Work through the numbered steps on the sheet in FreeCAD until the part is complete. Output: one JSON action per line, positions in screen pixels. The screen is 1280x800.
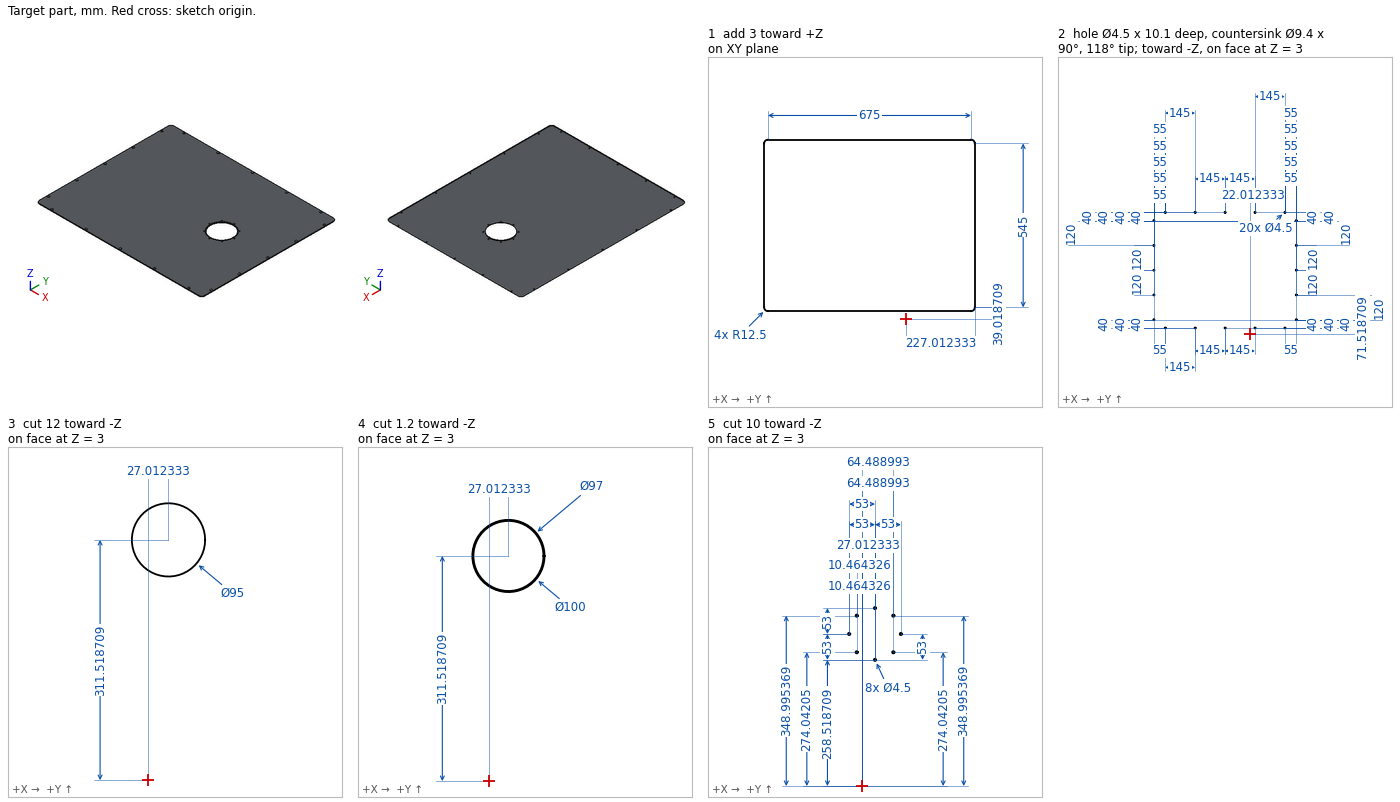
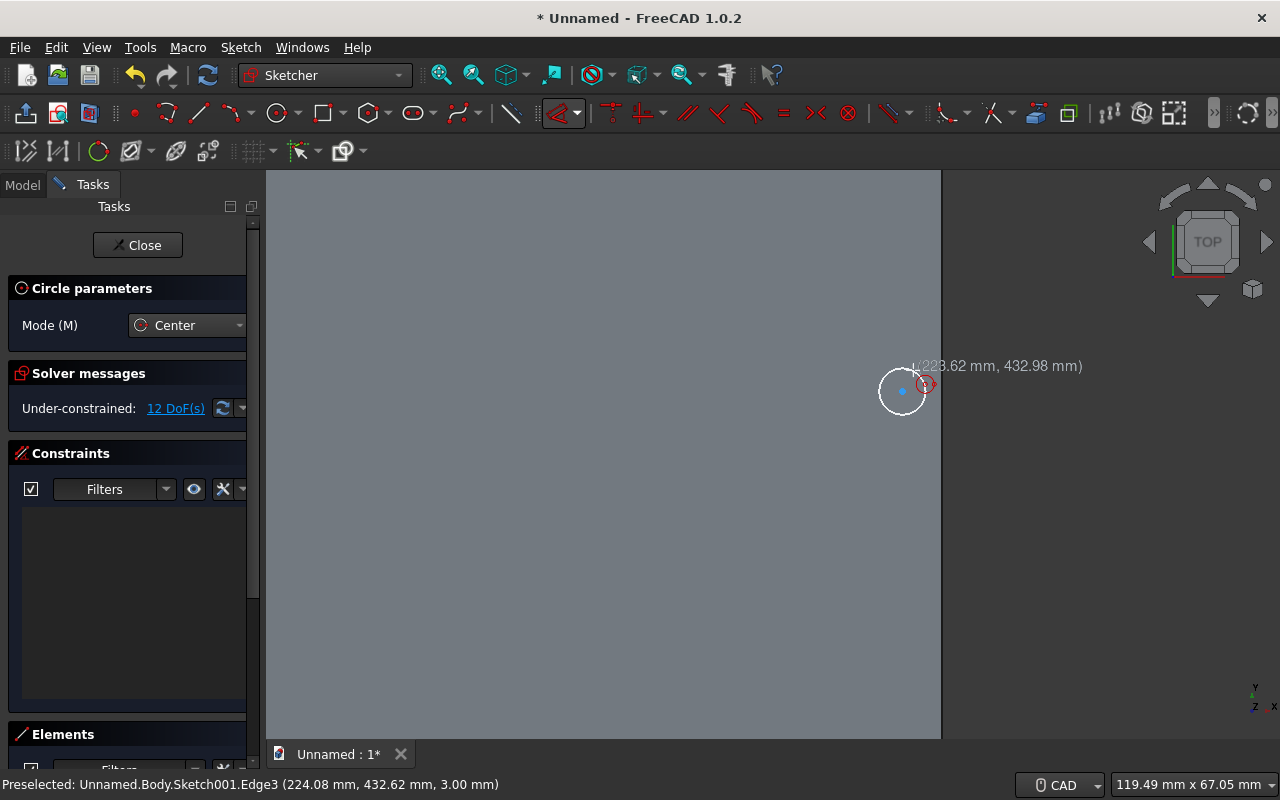
{"action": "scroll", "coordinate": [924, 369], "scroll_direction": "down", "scroll_amount": 13}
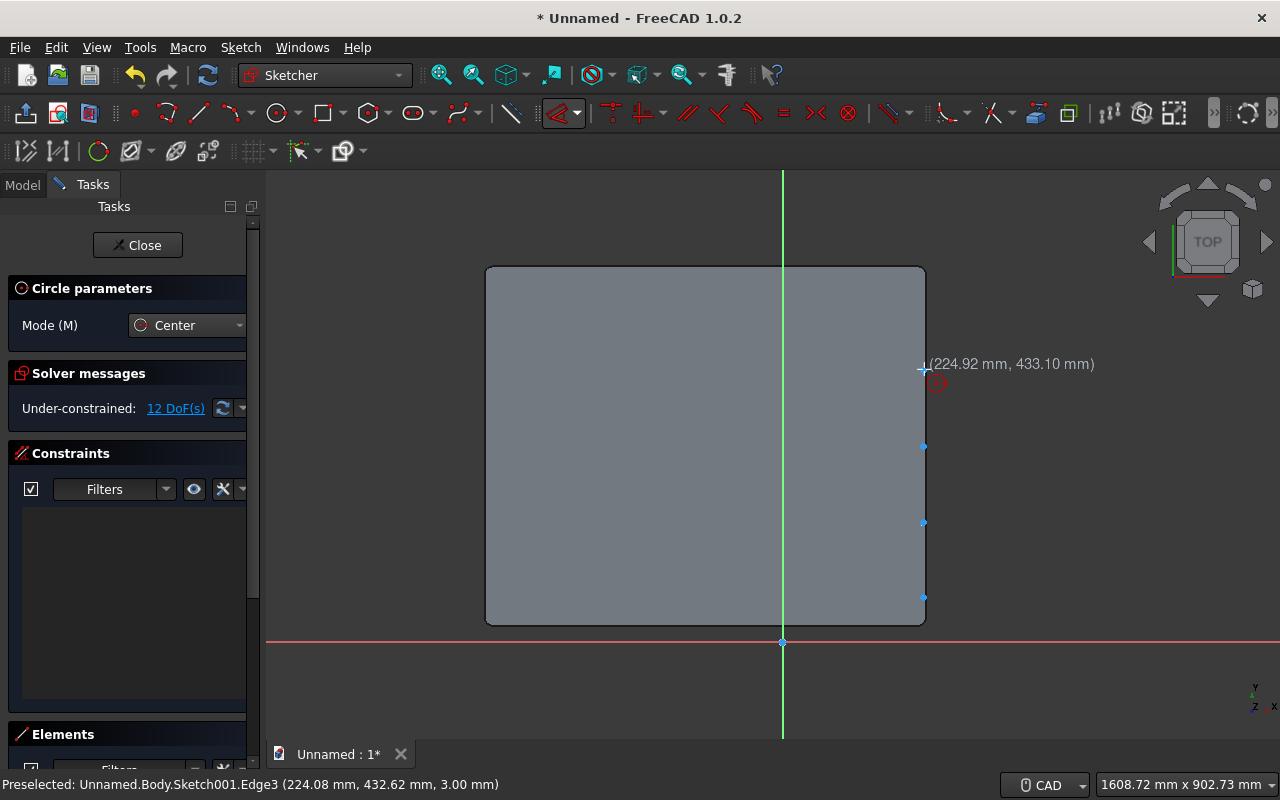
{"action": "scroll", "coordinate": [923, 295], "scroll_direction": "up", "scroll_amount": 14}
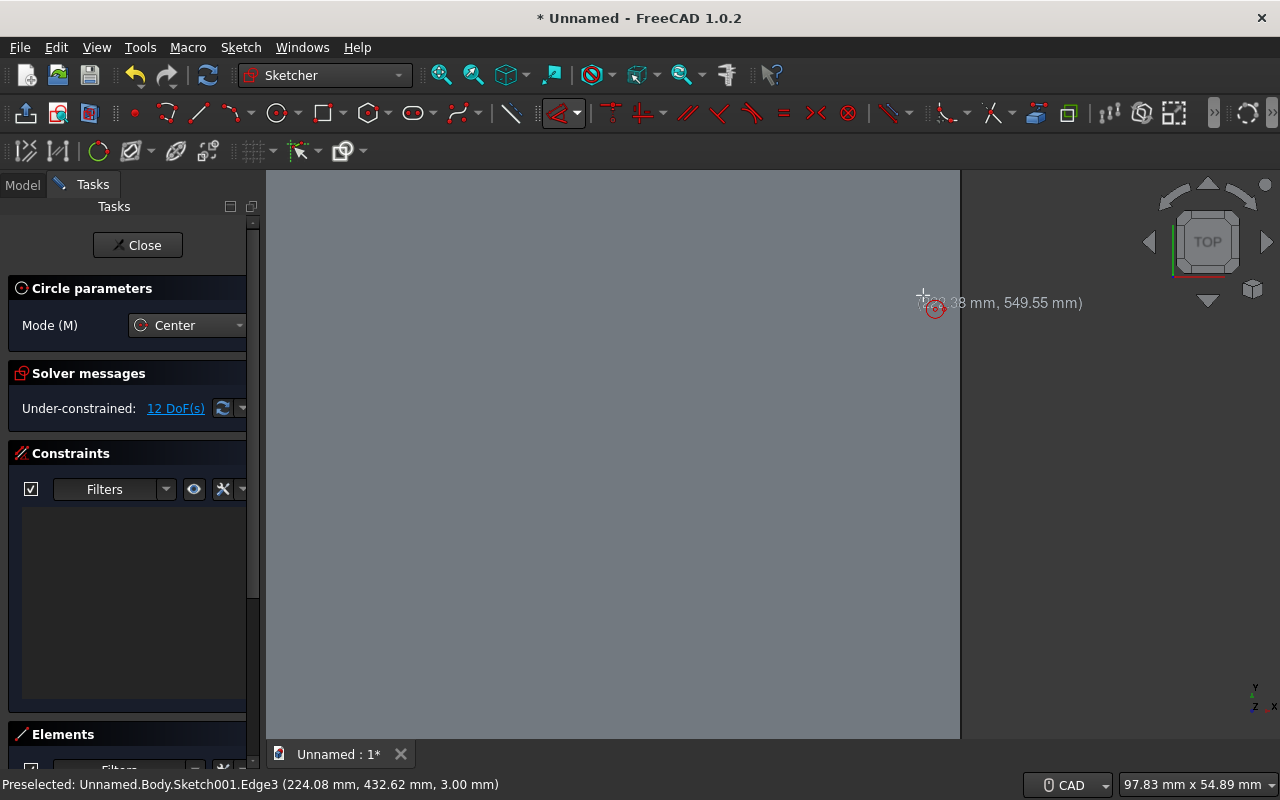
{"action": "scroll", "coordinate": [923, 294], "scroll_direction": "down", "scroll_amount": 14}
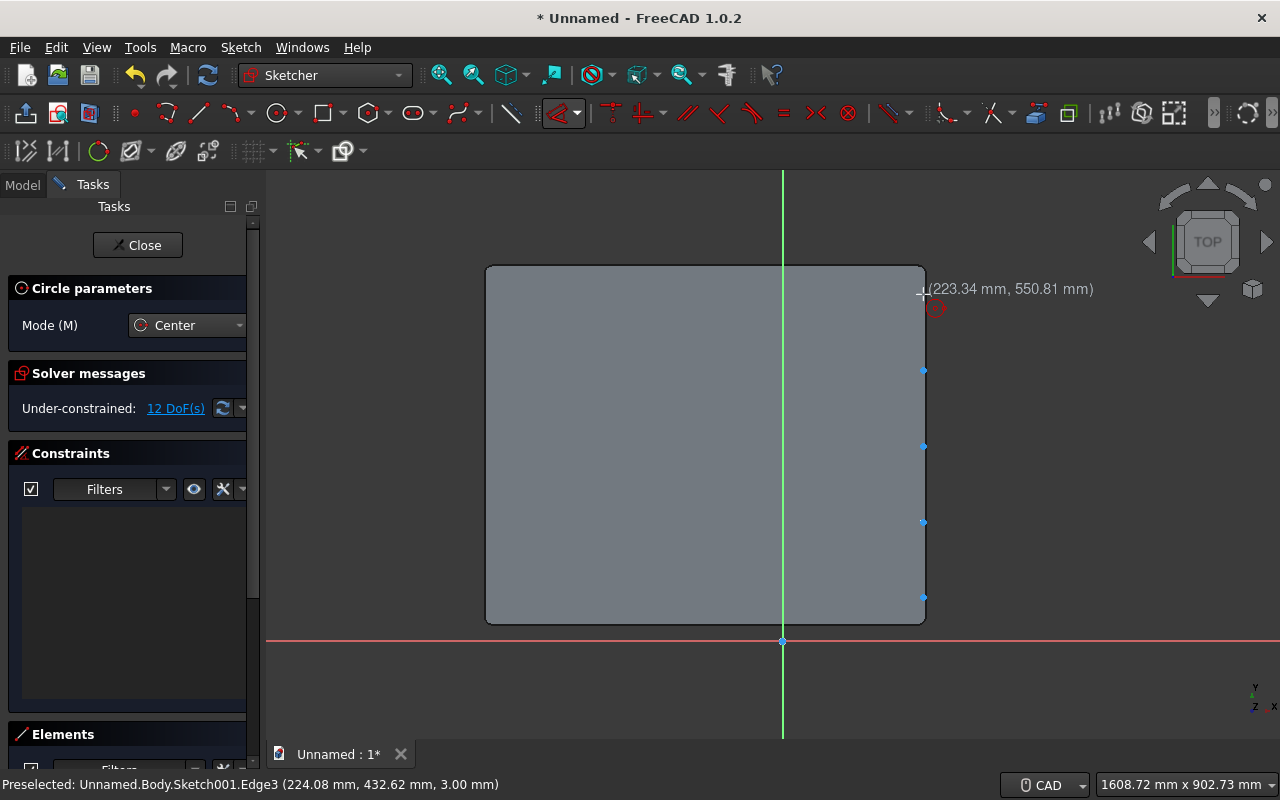
{"action": "left_click", "coordinate": [923, 294]}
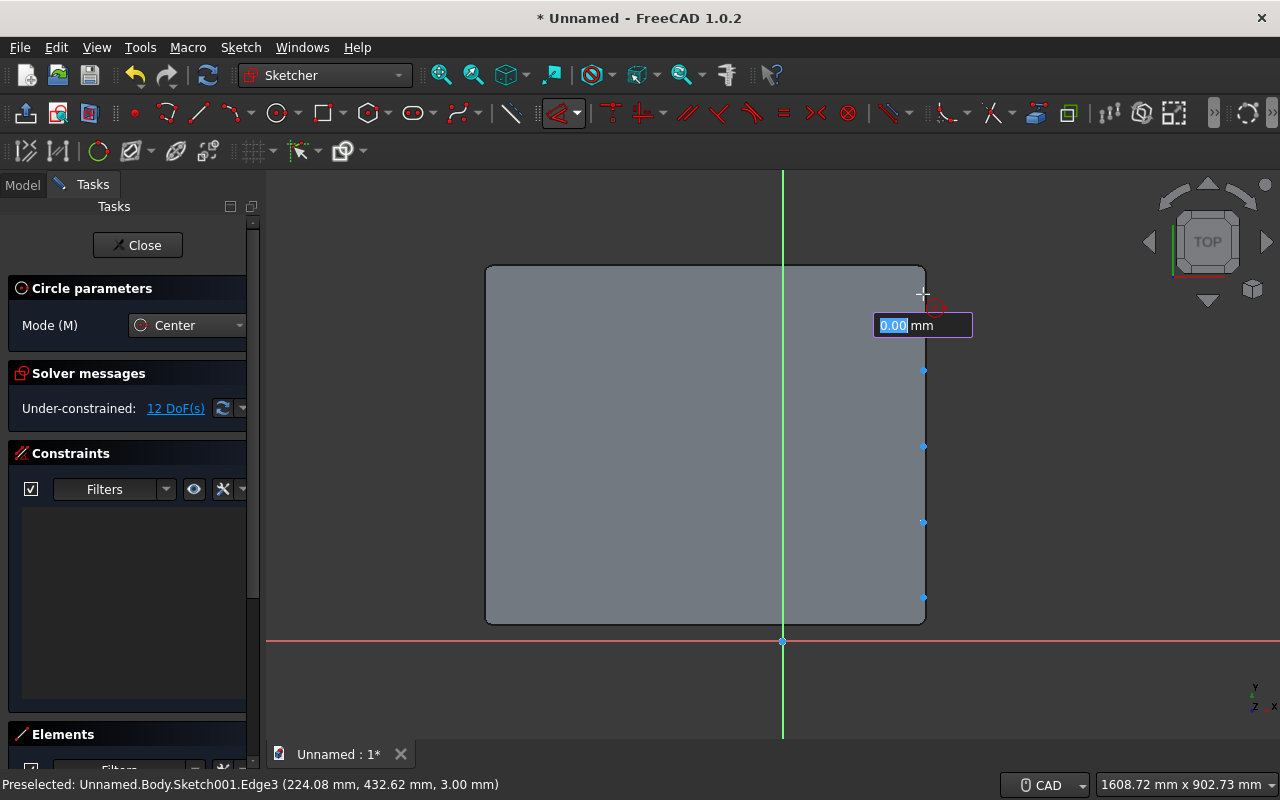
{"action": "scroll", "coordinate": [924, 293], "scroll_direction": "up", "scroll_amount": 13}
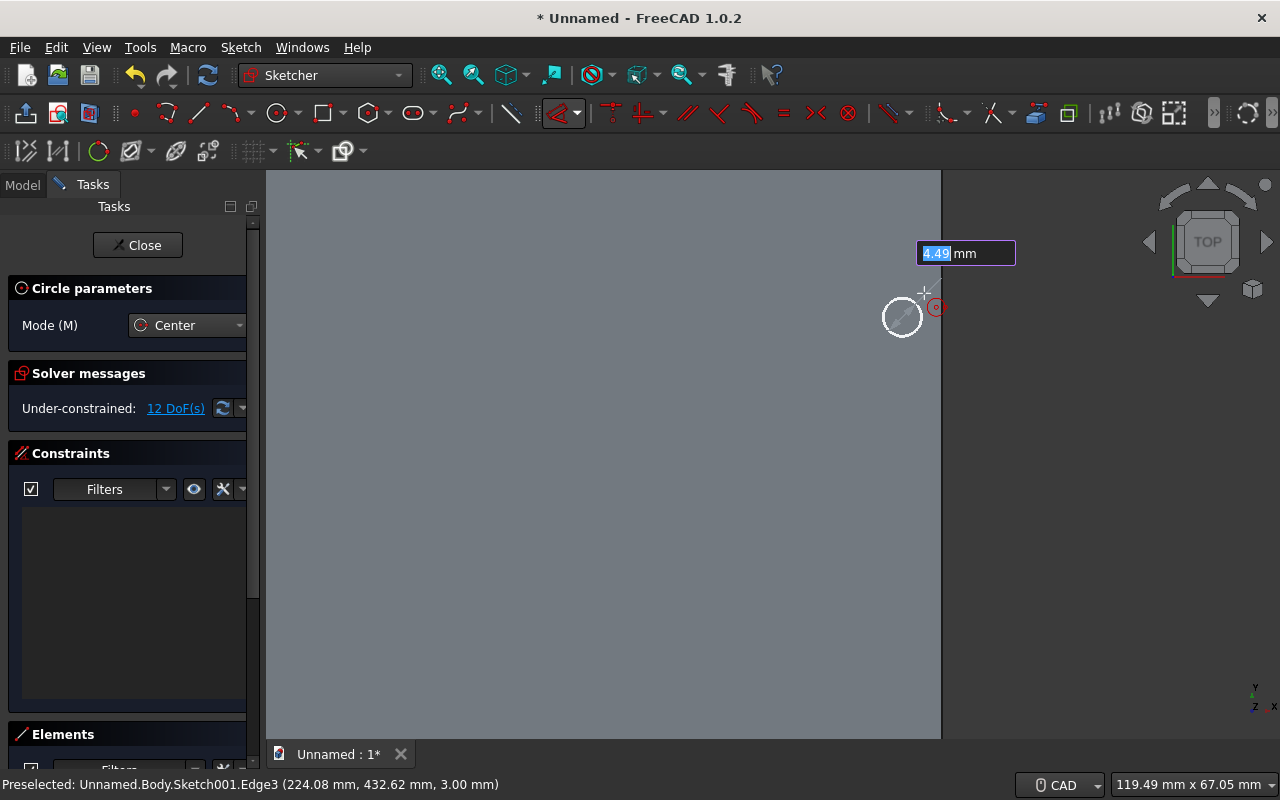
{"action": "left_click", "coordinate": [913, 288]}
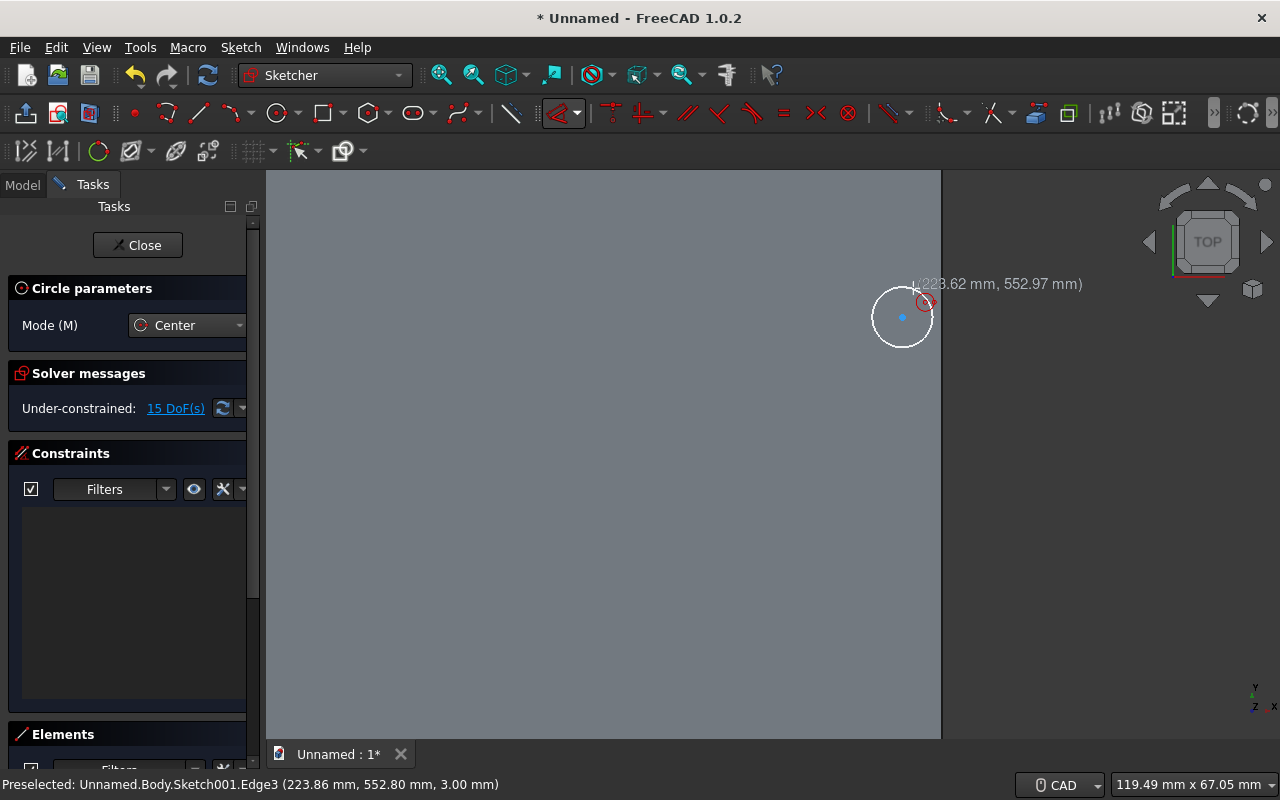
{"action": "scroll", "coordinate": [924, 293], "scroll_direction": "down", "scroll_amount": 13}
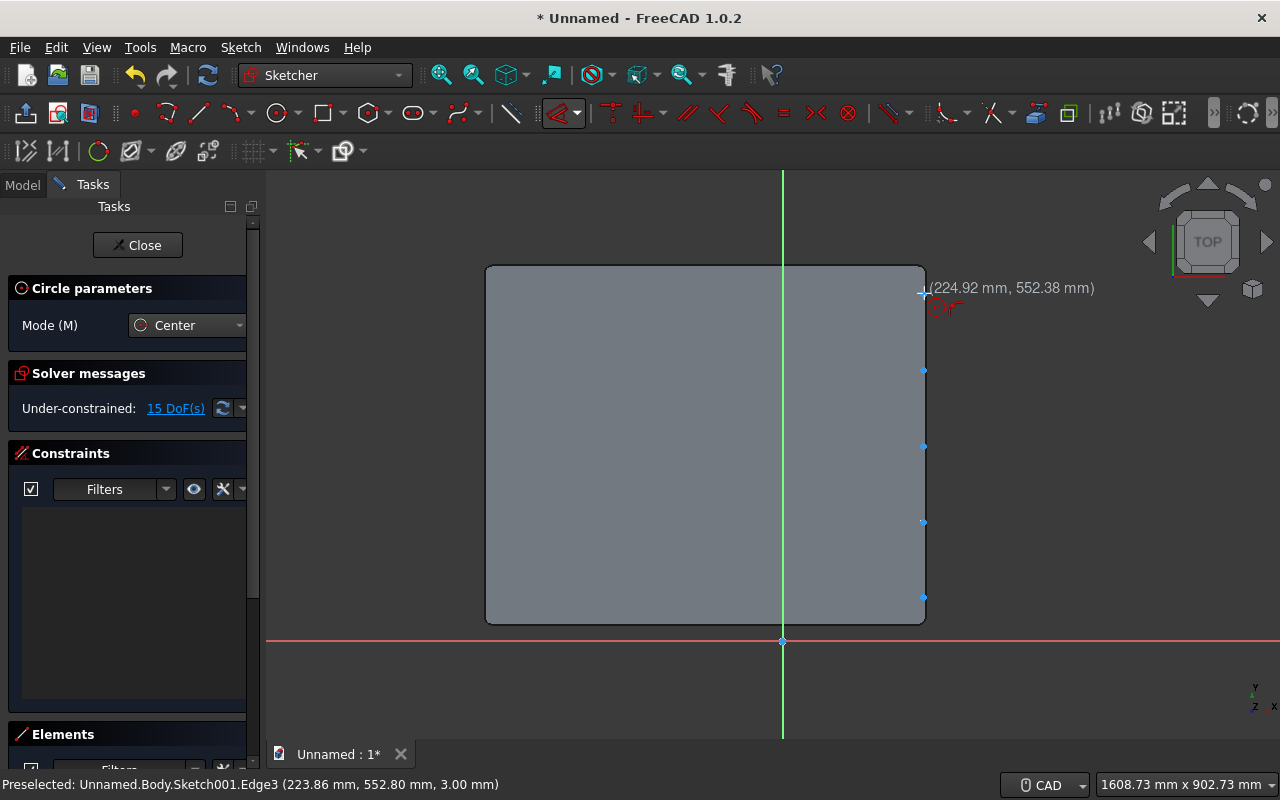
{"action": "scroll", "coordinate": [888, 269], "scroll_direction": "up", "scroll_amount": 14}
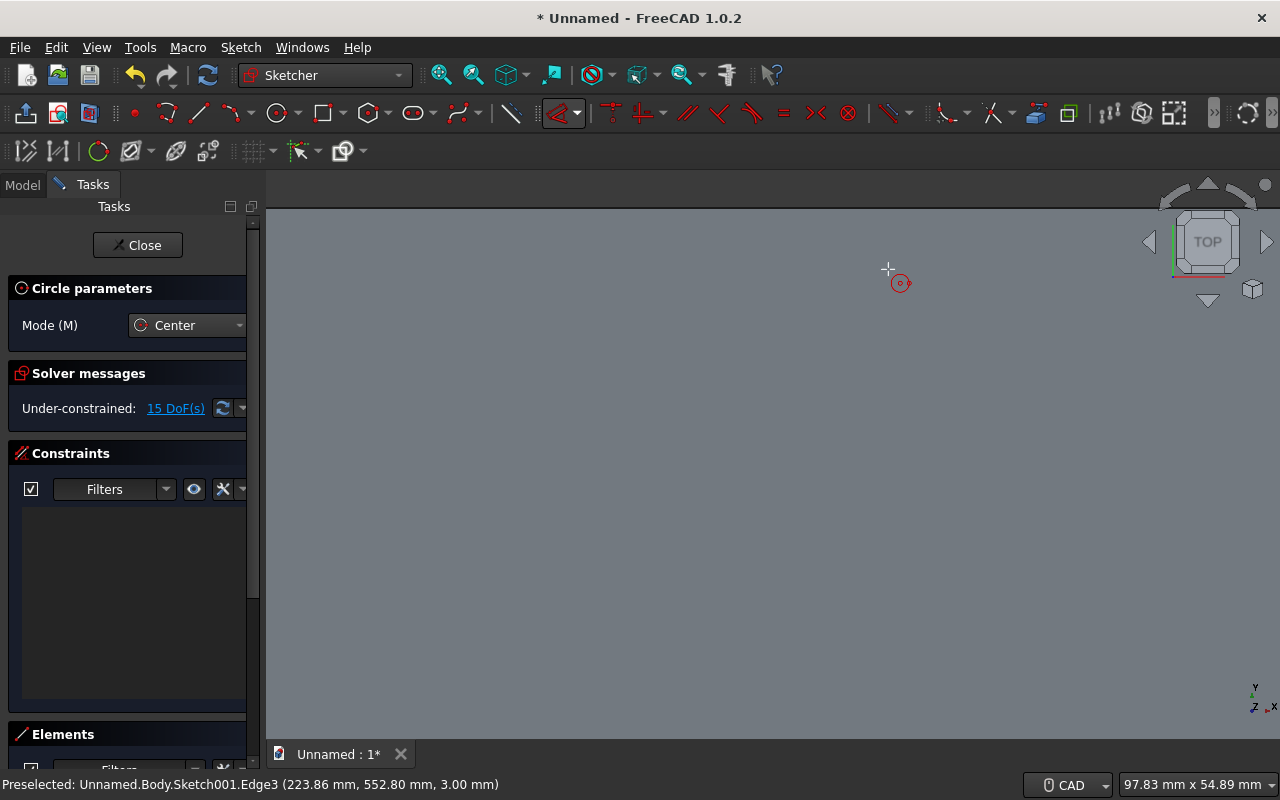
{"action": "scroll", "coordinate": [888, 269], "scroll_direction": "down", "scroll_amount": 14}